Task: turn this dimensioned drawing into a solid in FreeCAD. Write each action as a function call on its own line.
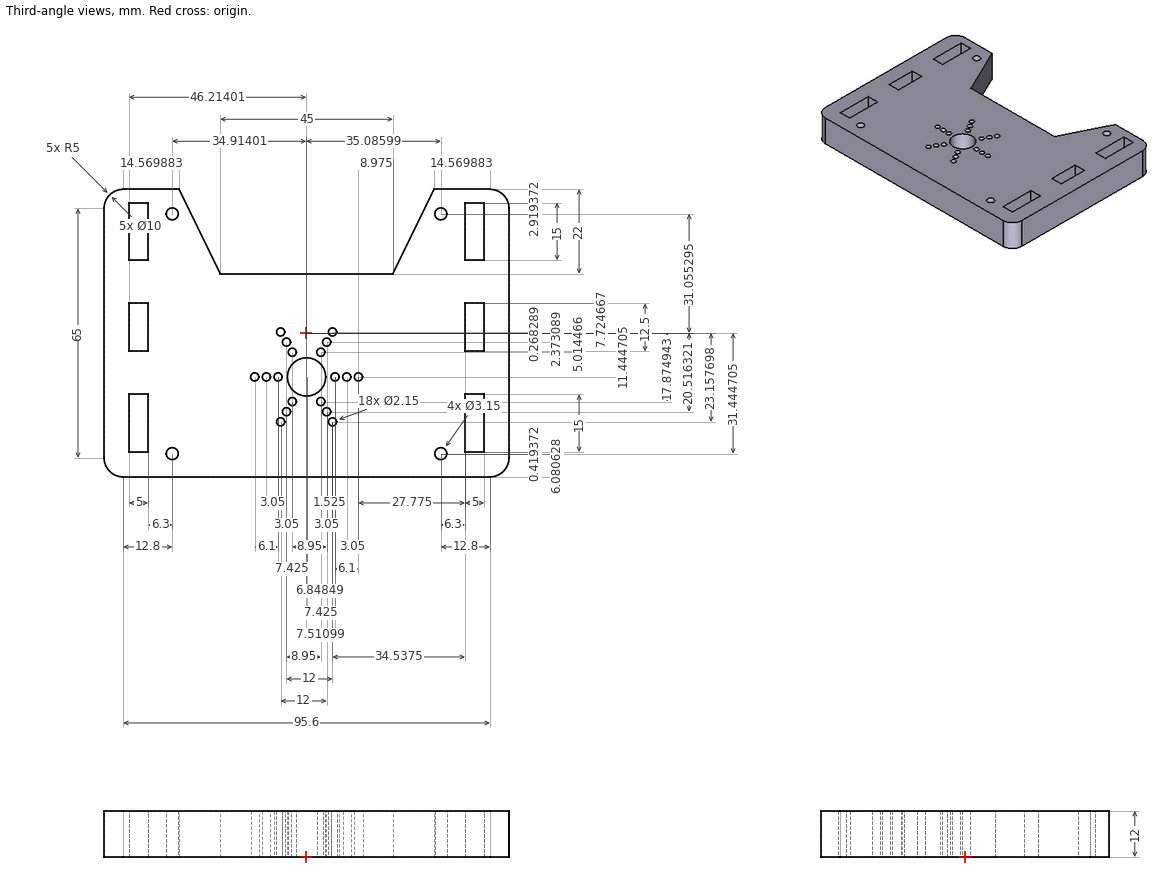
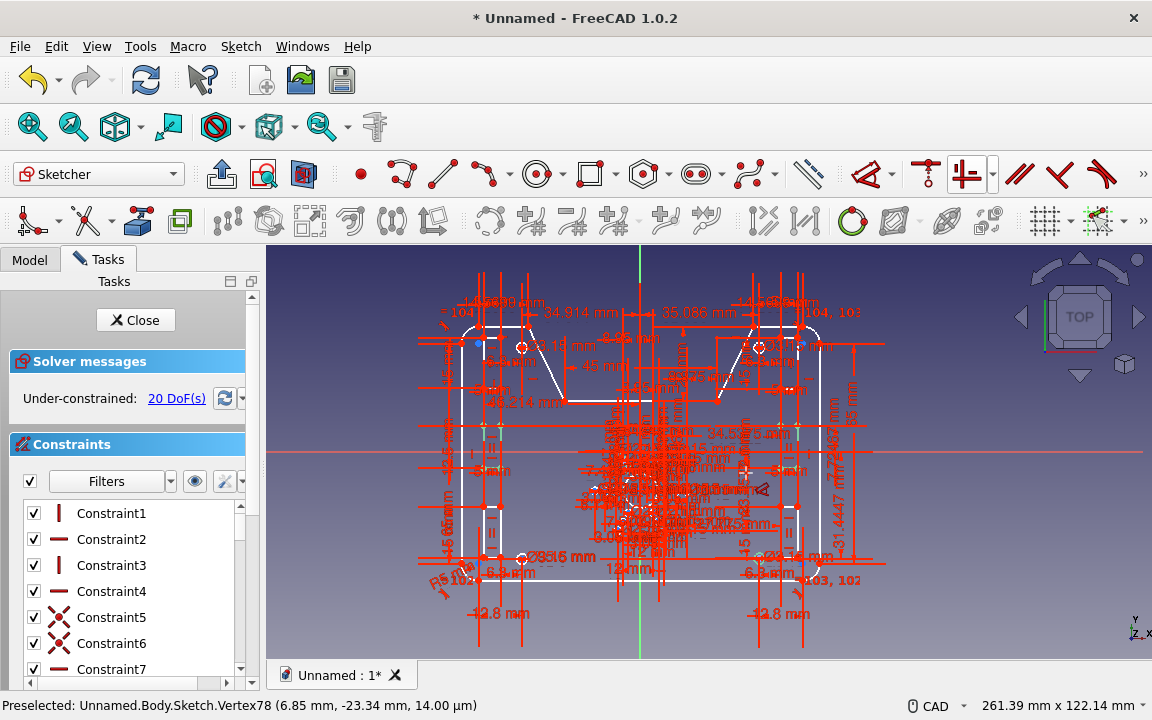
click(659, 522)
click(765, 503)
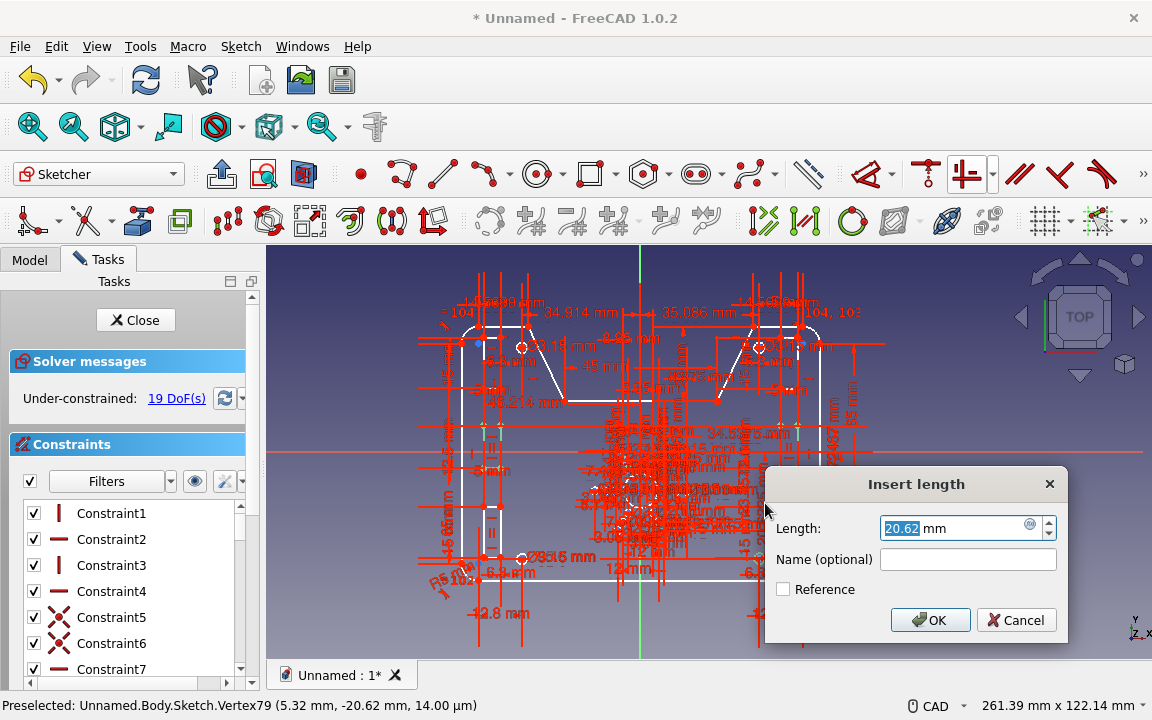
text(20.516321)
key(Return)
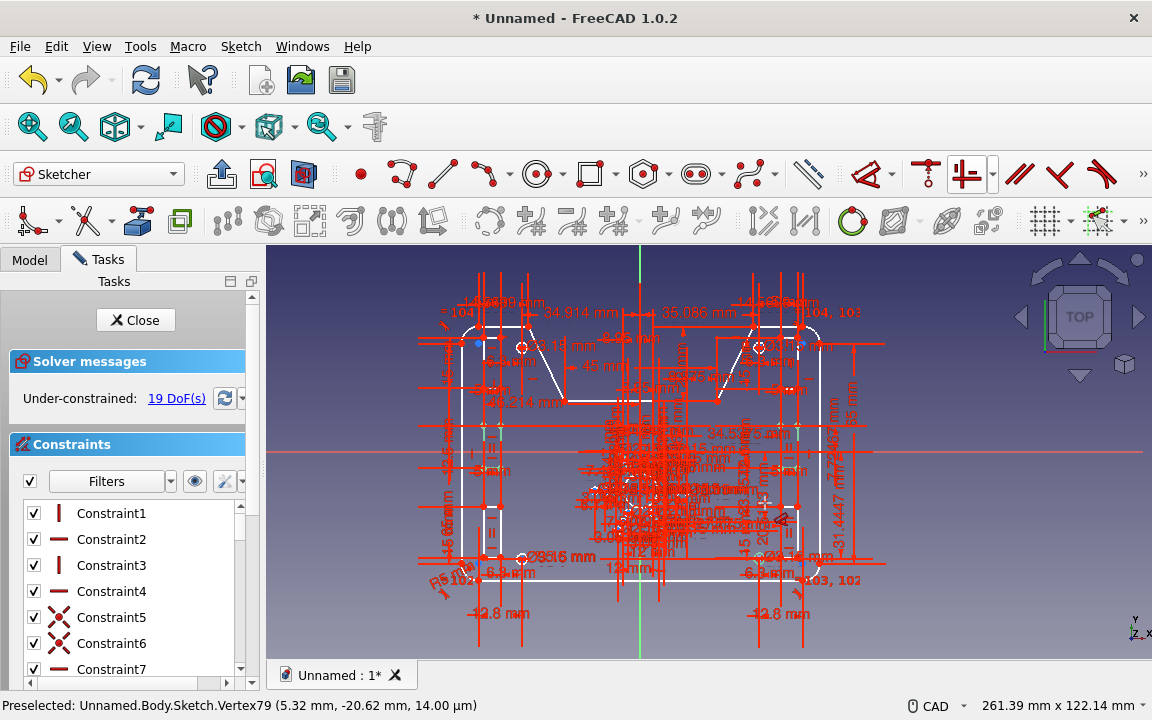
scroll(653, 513, up, 2)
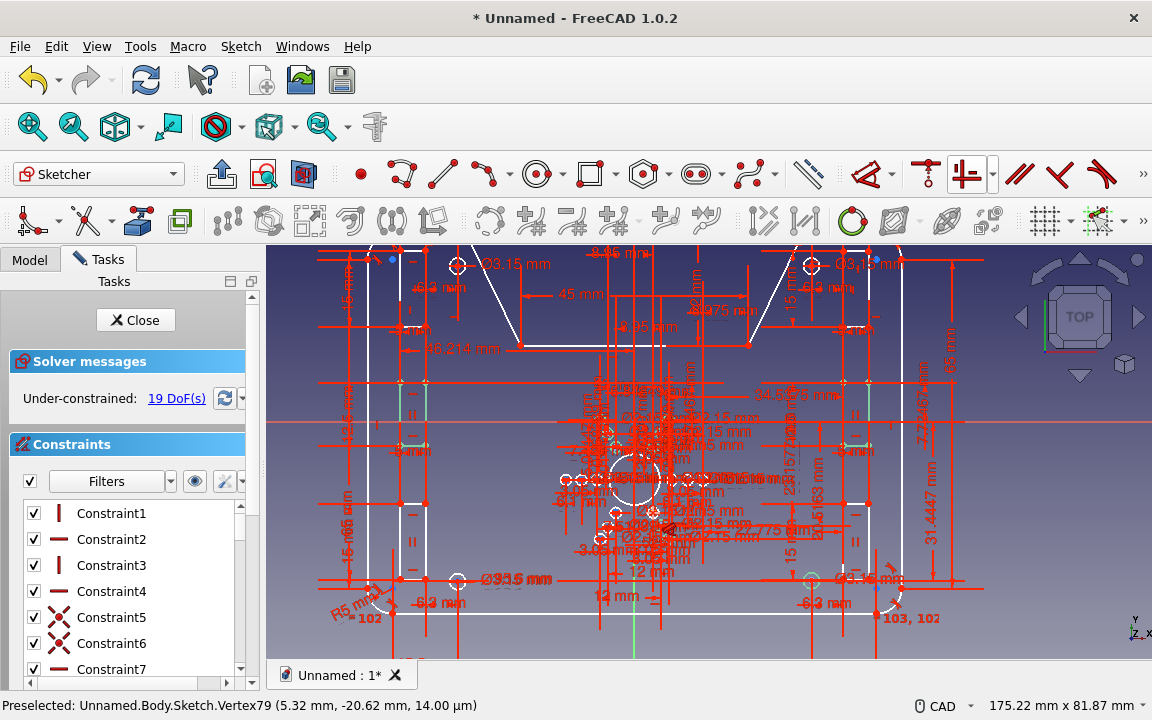
click(653, 513)
click(528, 467)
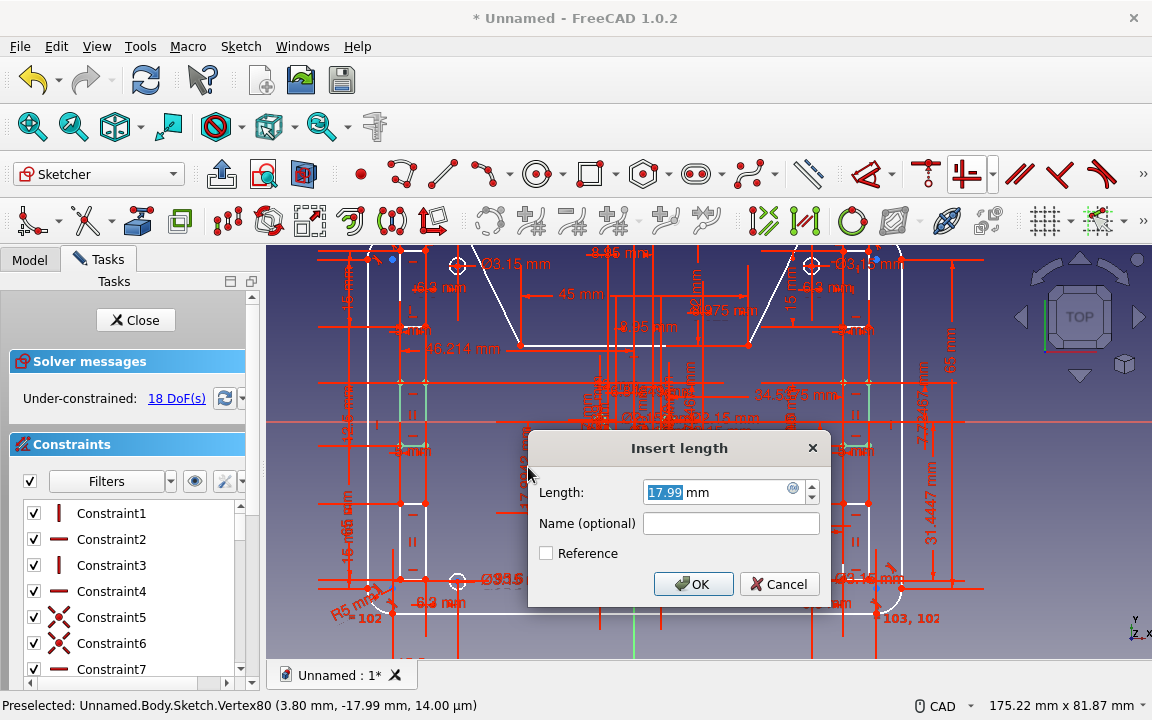
text(17.874943)
key(Return)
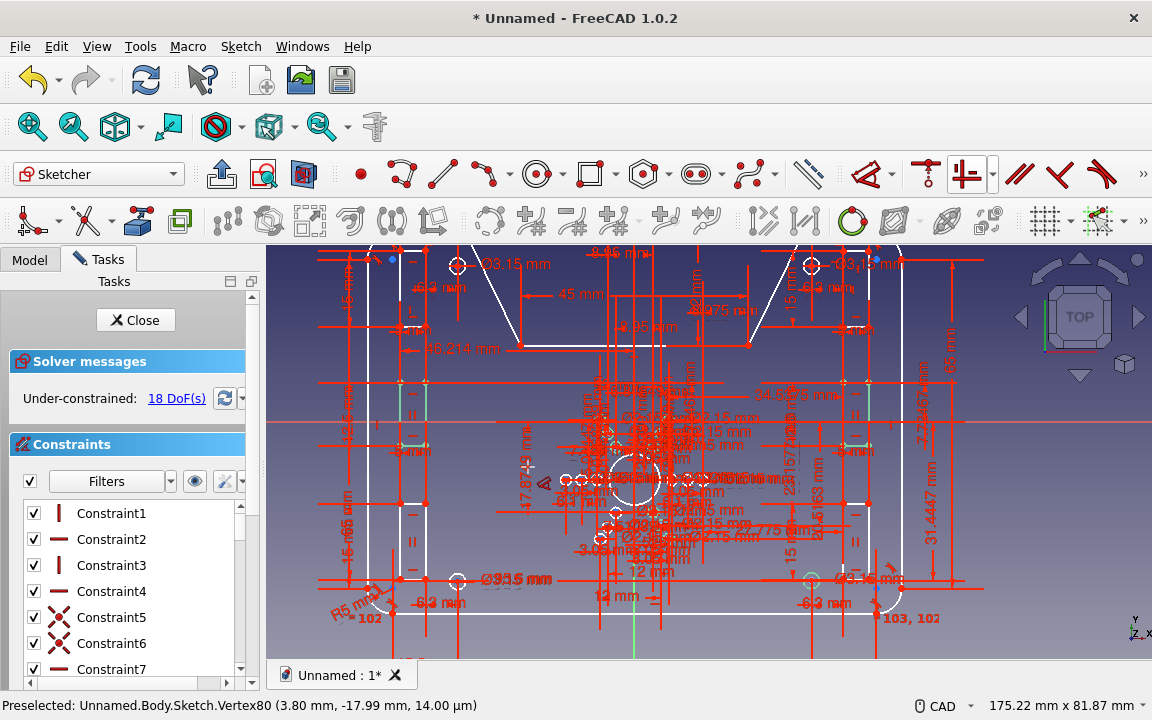
click(703, 481)
click(504, 438)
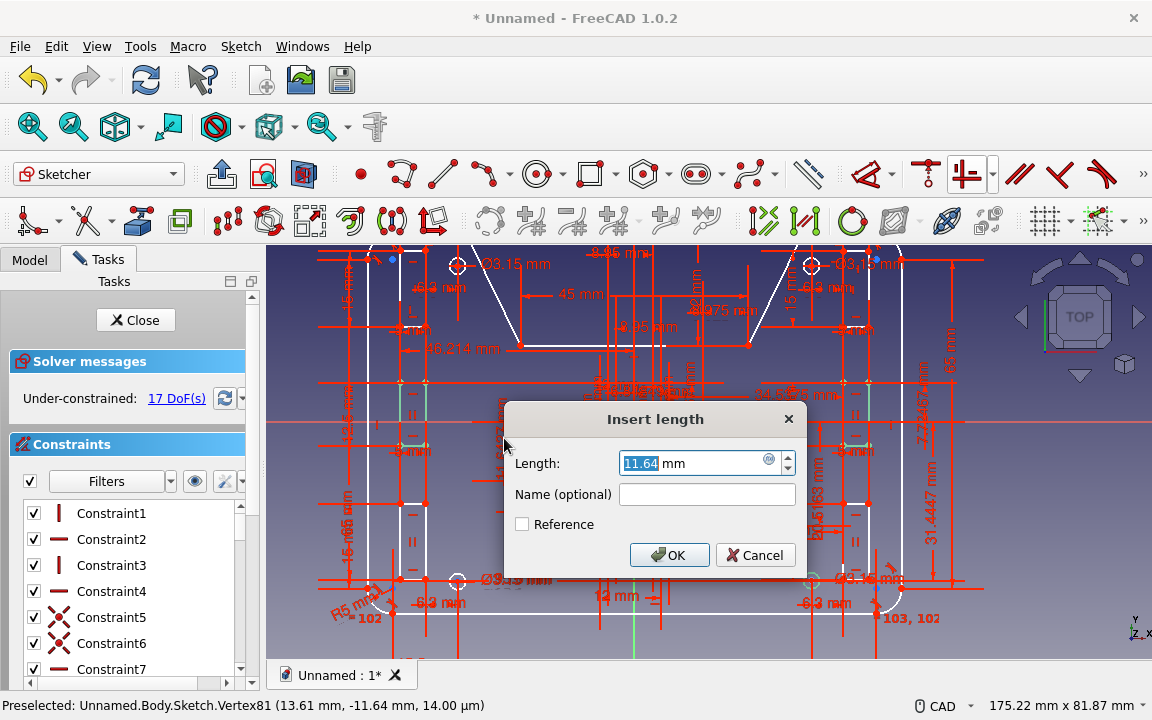
text(11.444705)
key(Return)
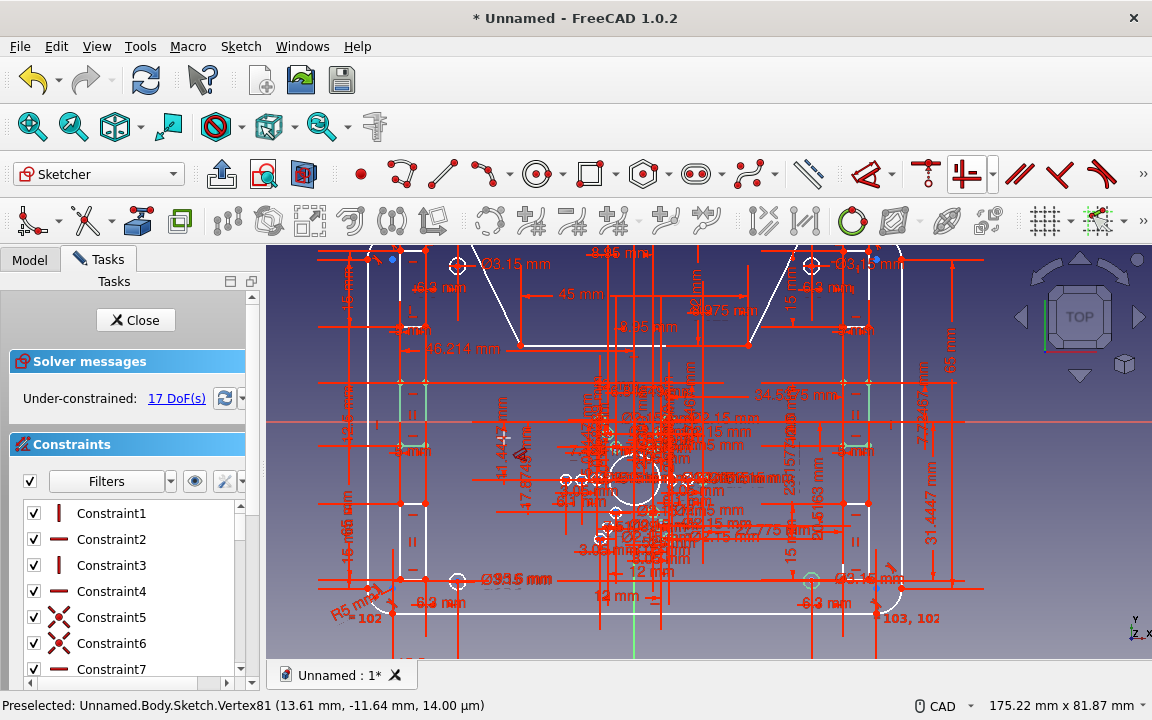
click(688, 480)
click(868, 464)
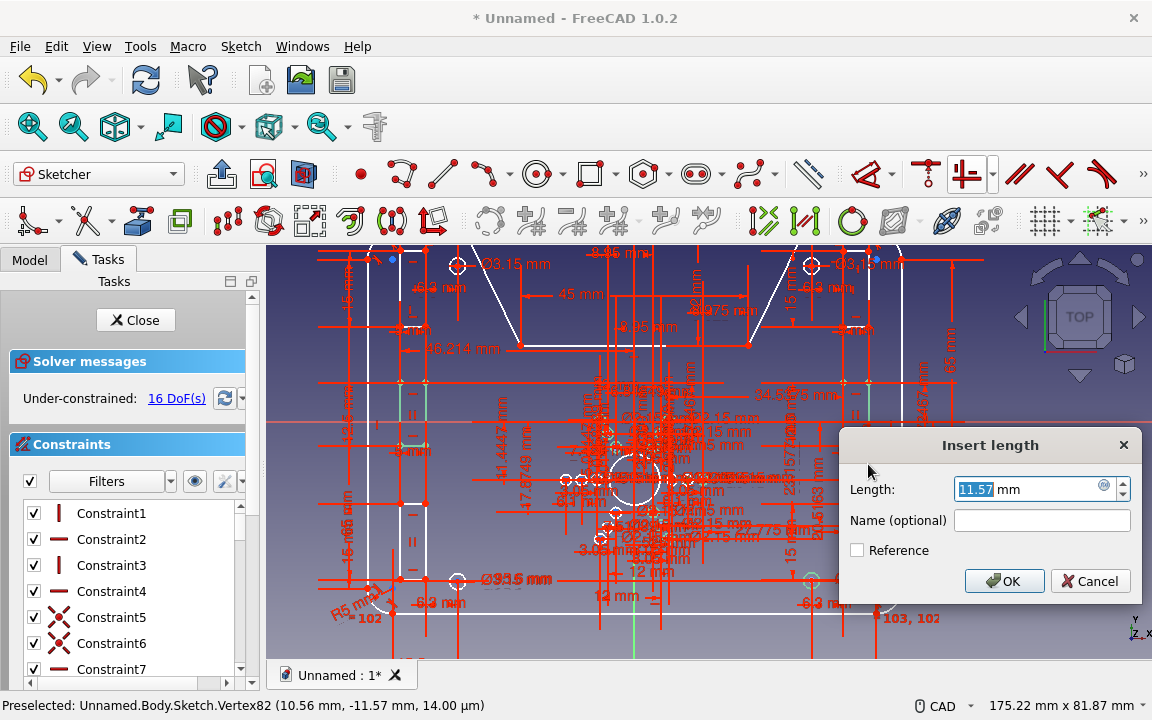
text(11.444705)
key(Return)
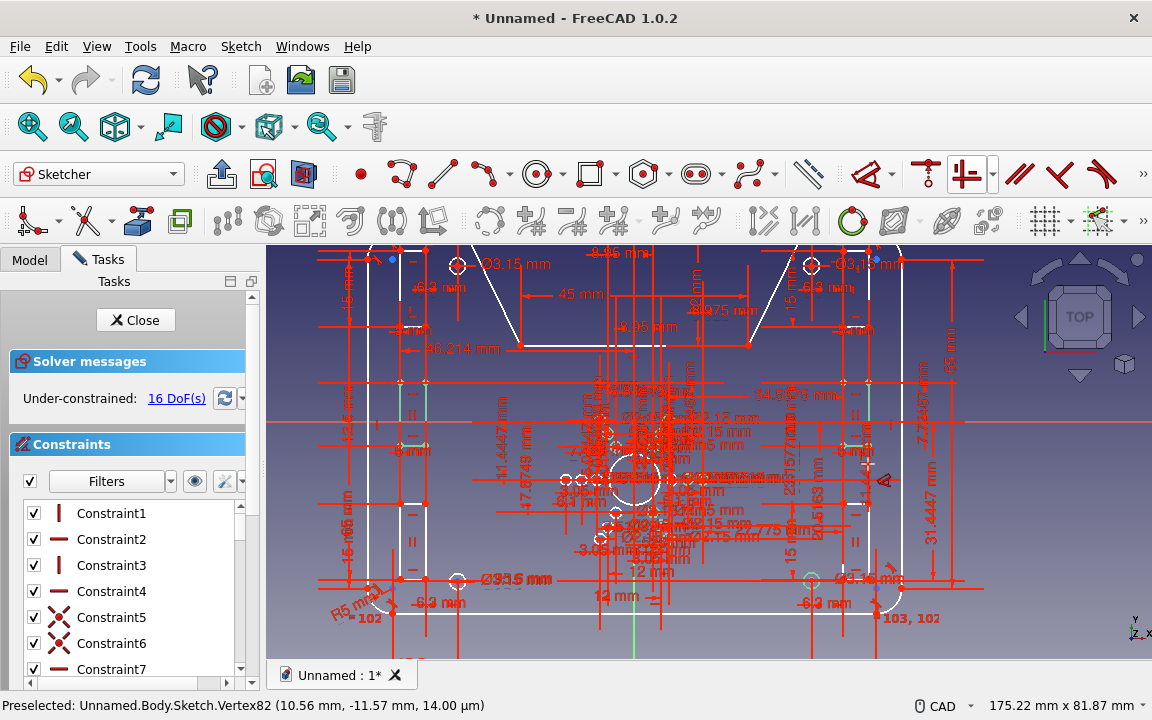
click(672, 480)
click(454, 464)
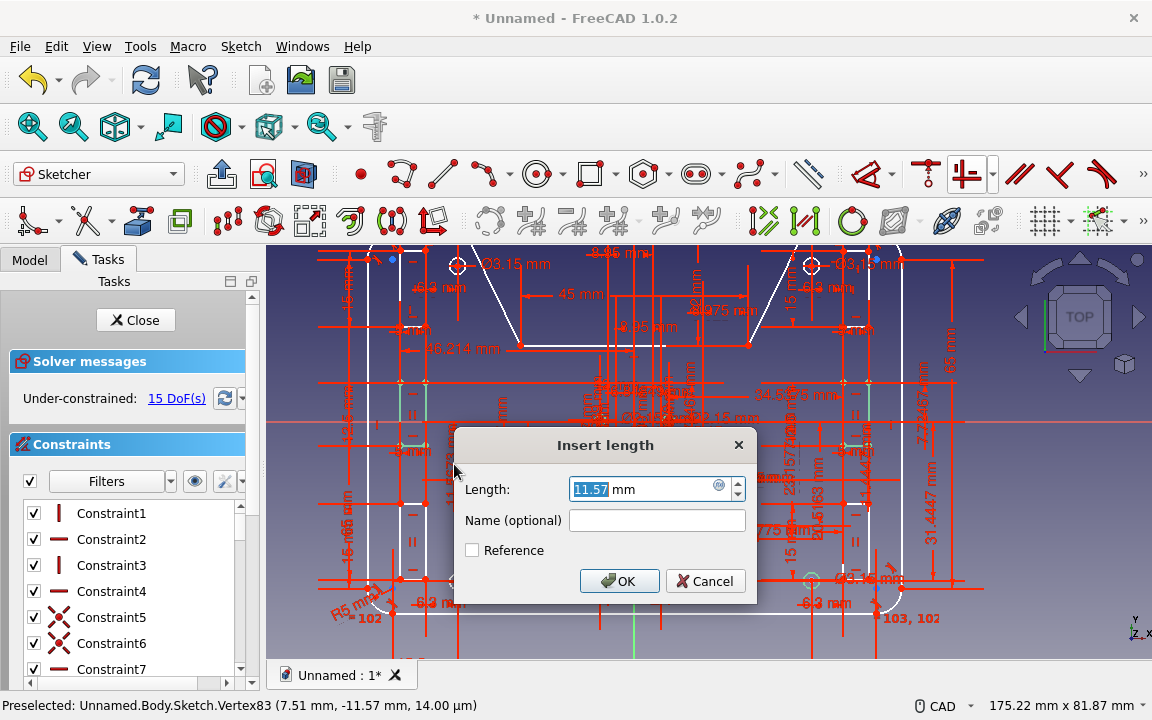
text(11.444705)
key(Return)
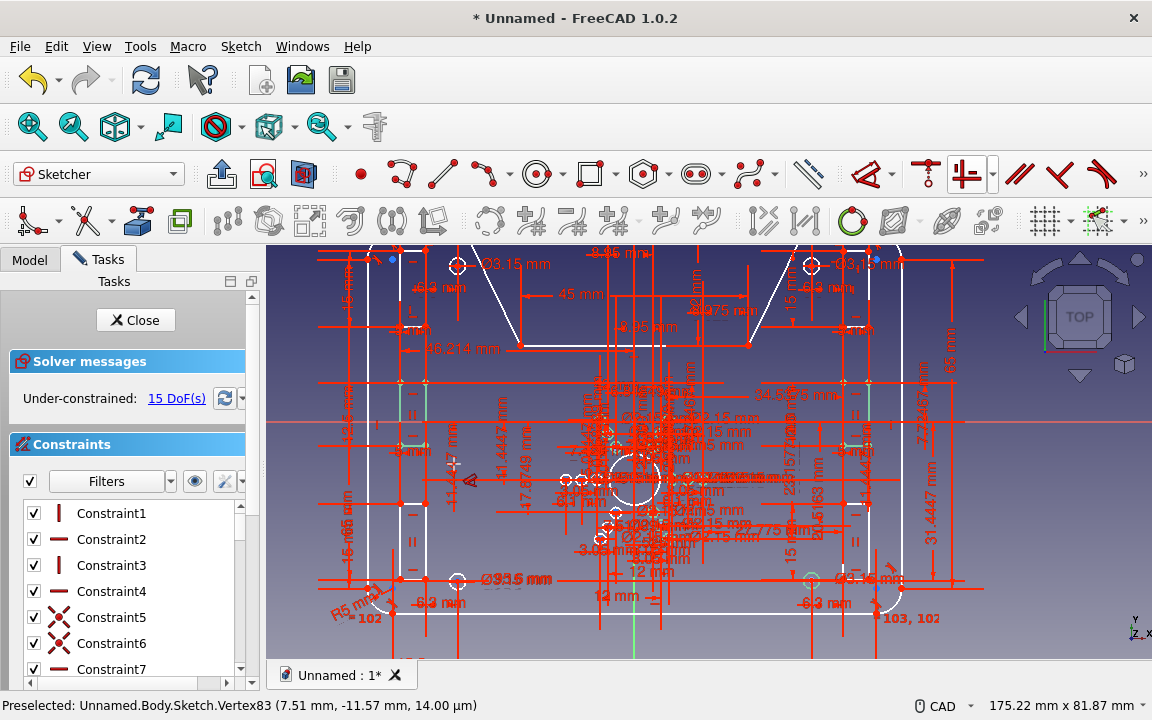
click(608, 527)
click(502, 499)